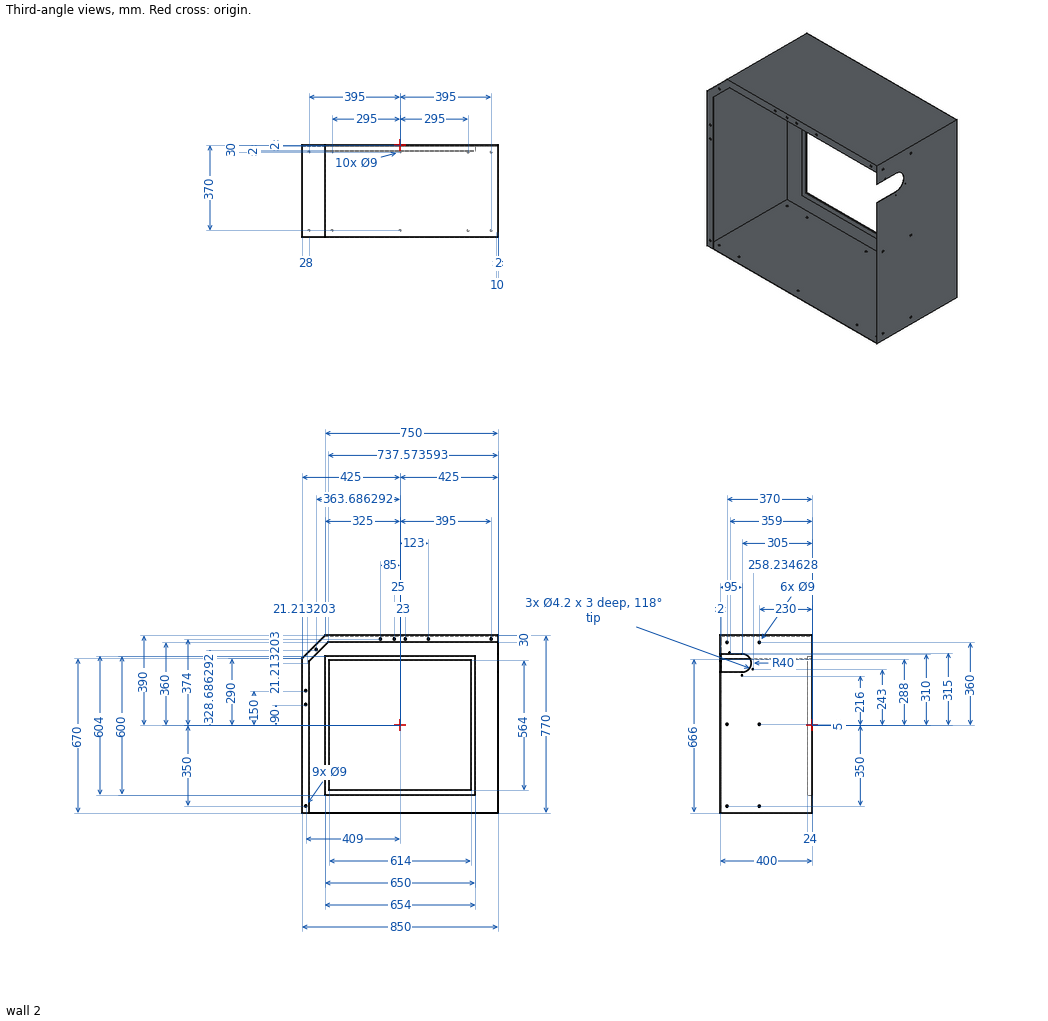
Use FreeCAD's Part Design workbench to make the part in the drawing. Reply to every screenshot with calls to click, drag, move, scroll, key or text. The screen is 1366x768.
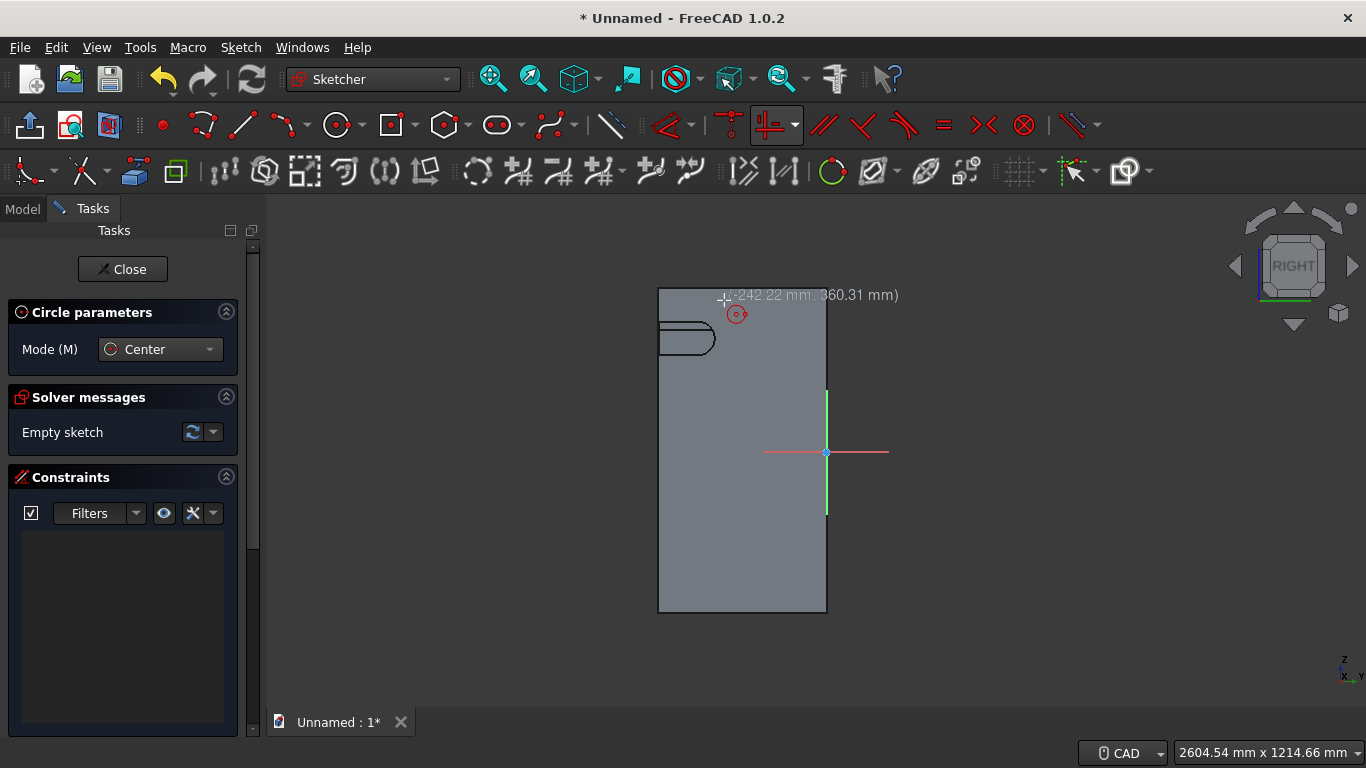
click(730, 300)
move(731, 299)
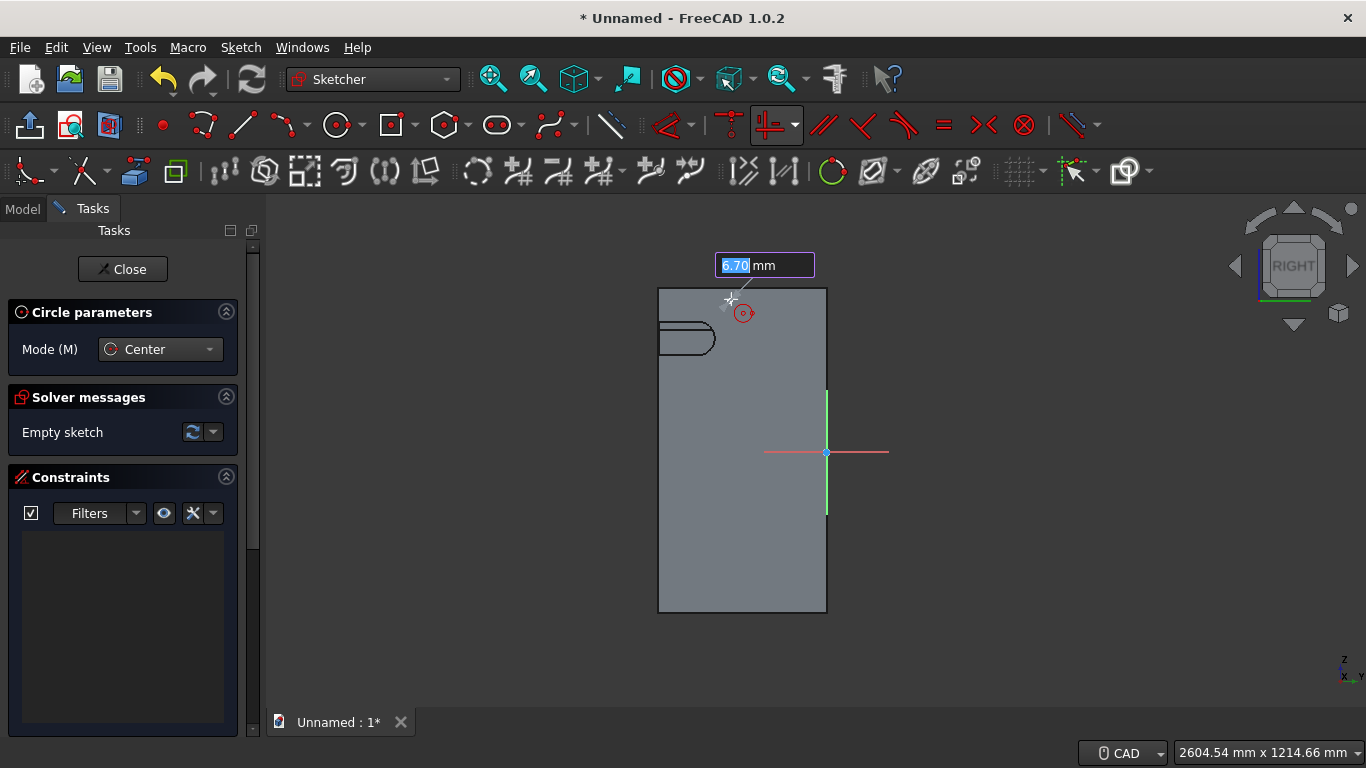
text(9)
key(Return)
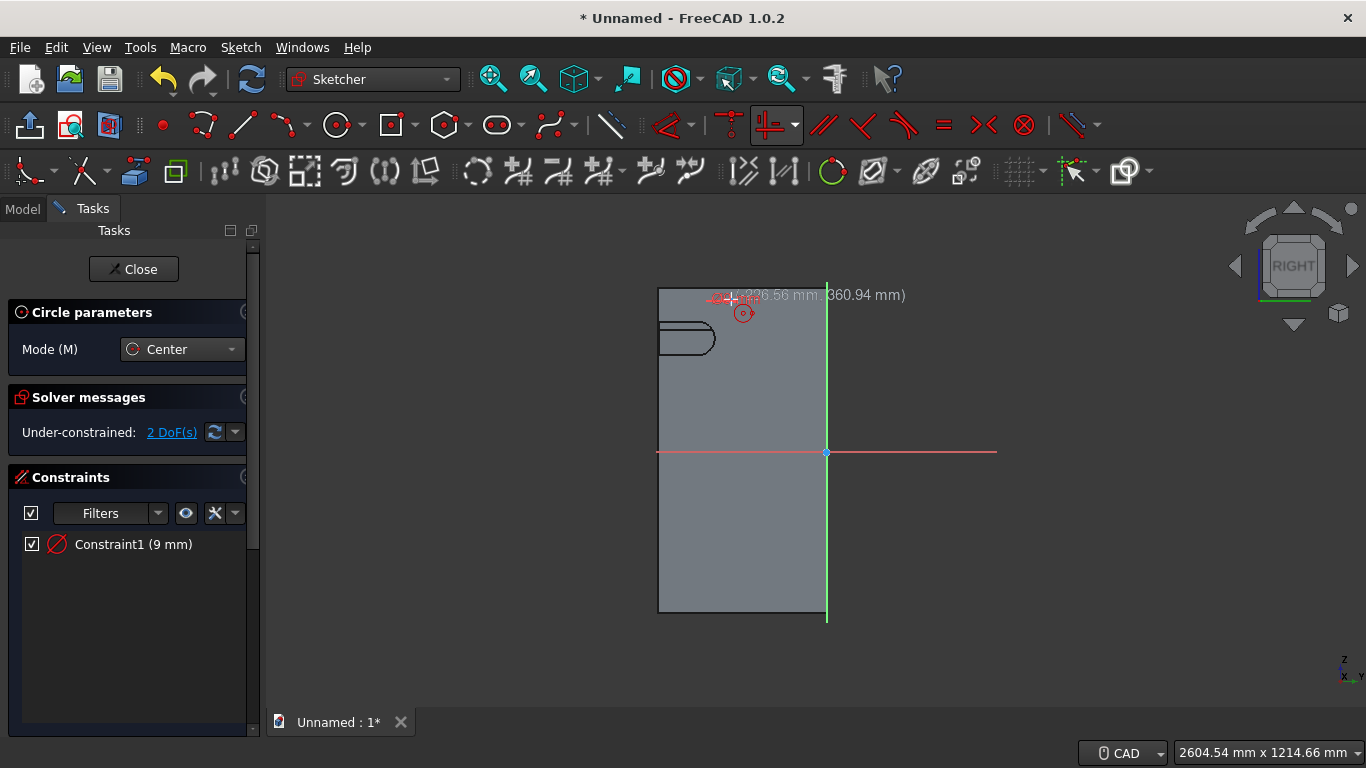
scroll(670, 300, up, 13)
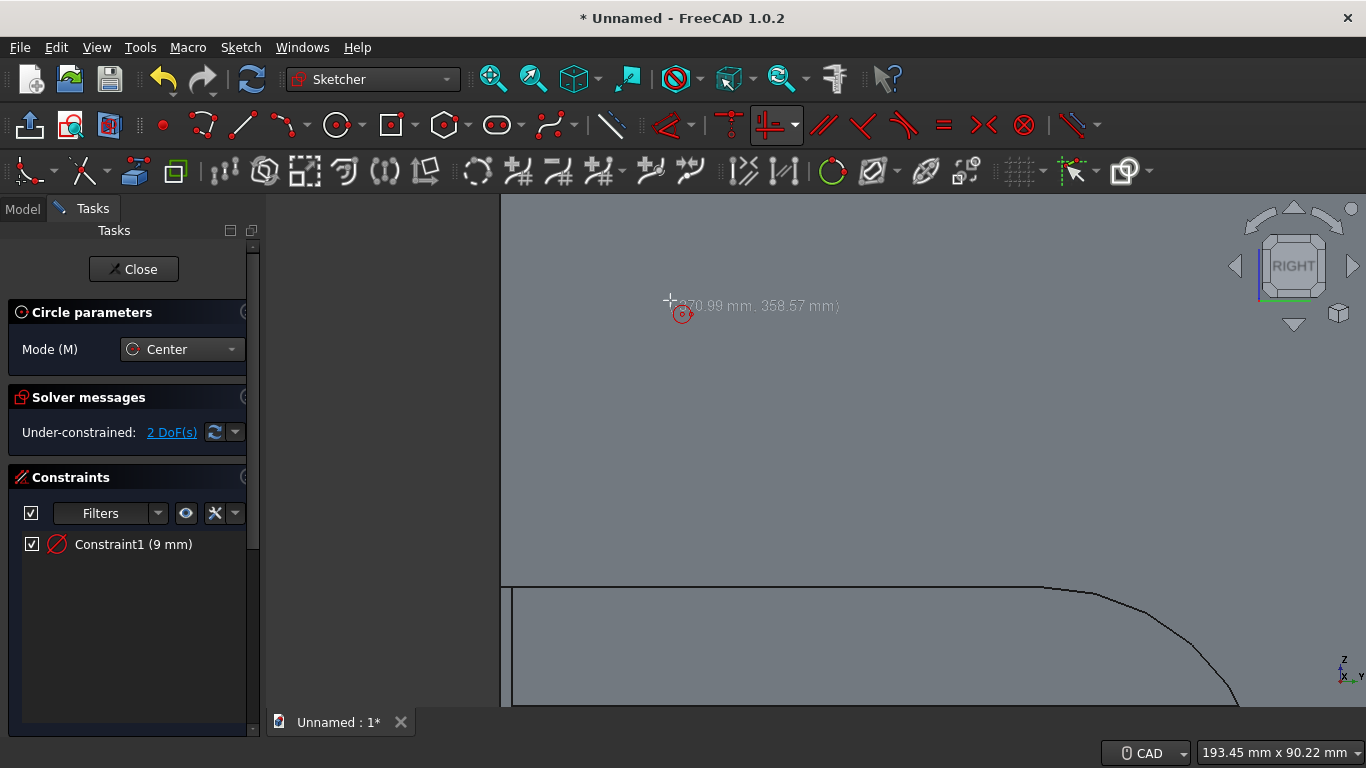
scroll(670, 300, down, 13)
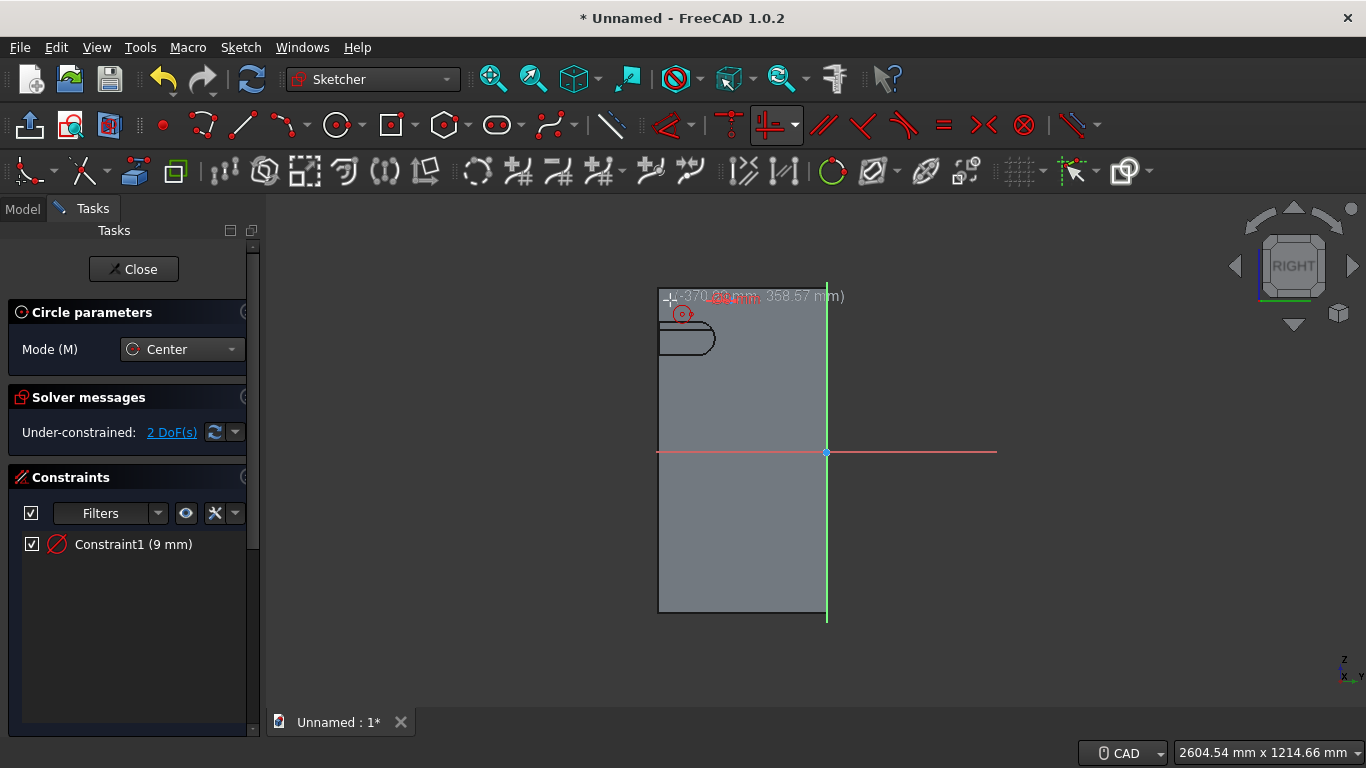
click(670, 300)
move(672, 299)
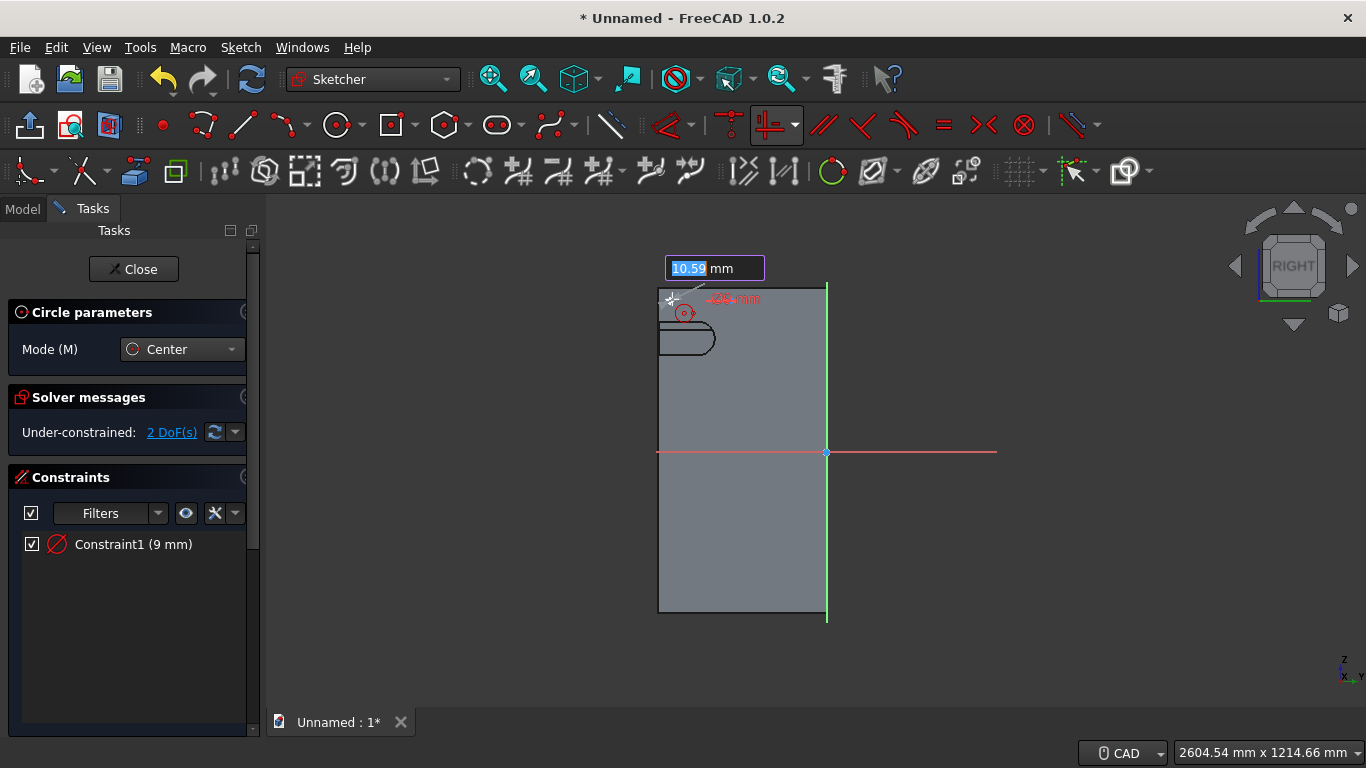
text(9)
key(Return)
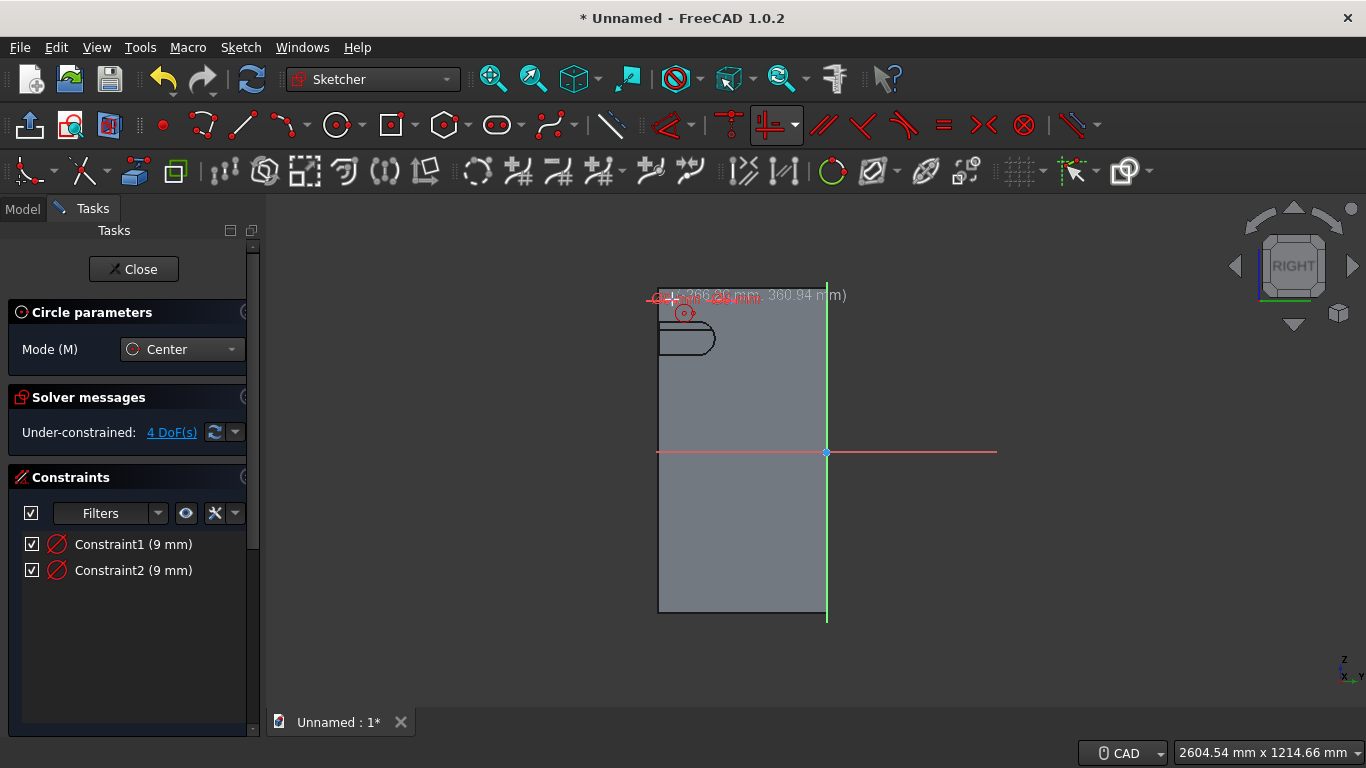
scroll(730, 450, up, 13)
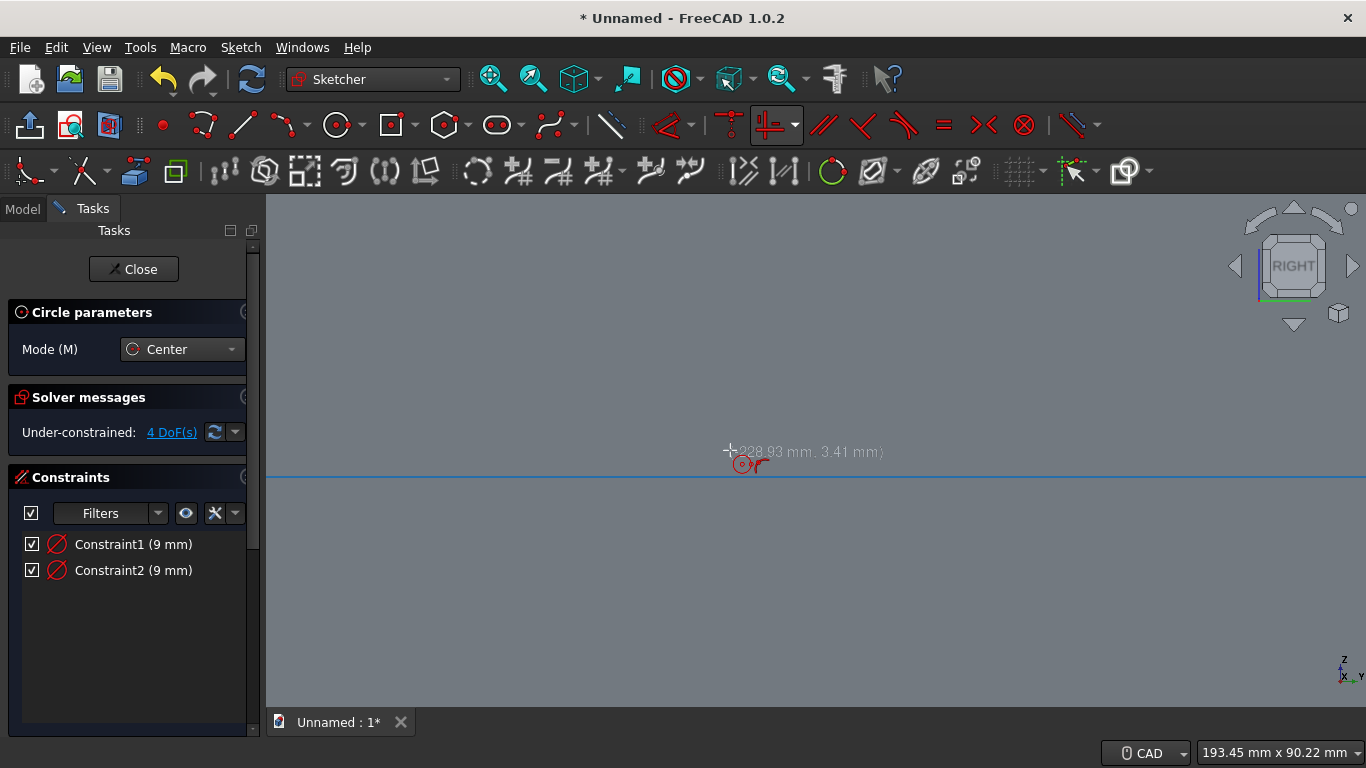
click(719, 448)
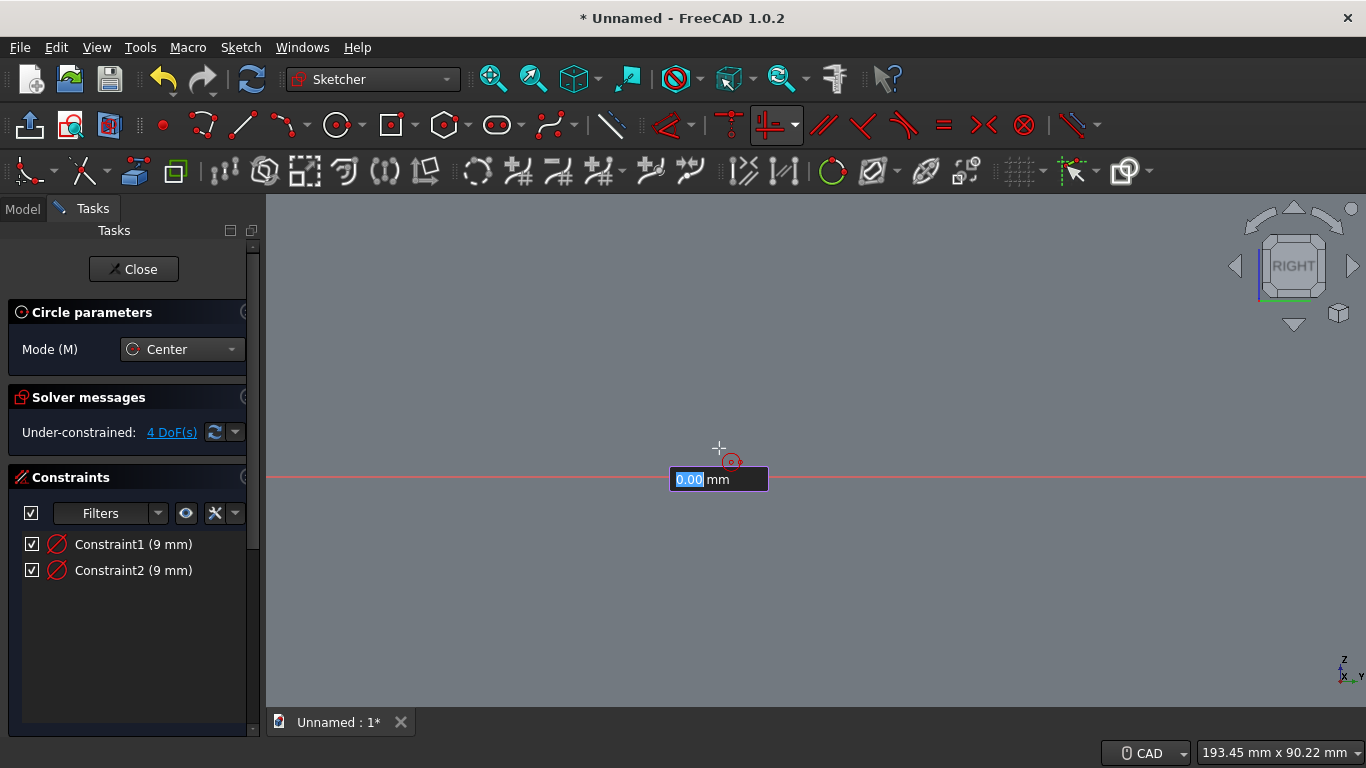
scroll(730, 451, down, 13)